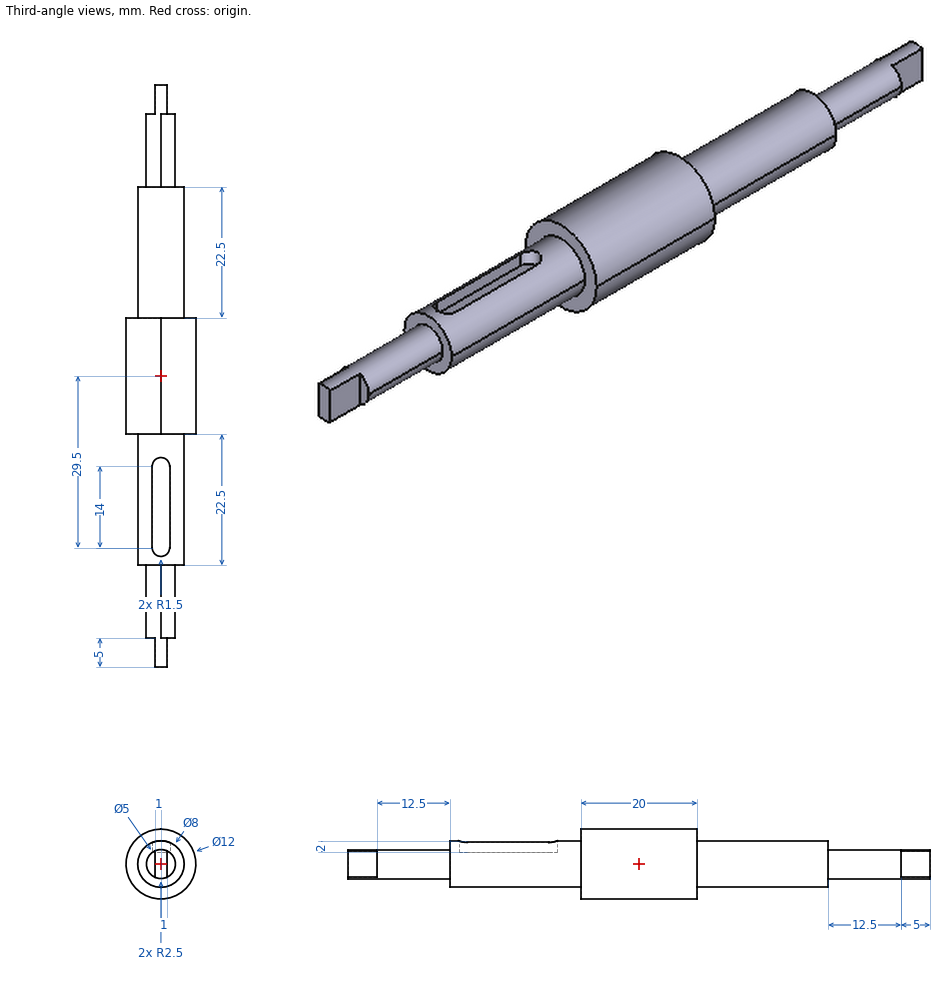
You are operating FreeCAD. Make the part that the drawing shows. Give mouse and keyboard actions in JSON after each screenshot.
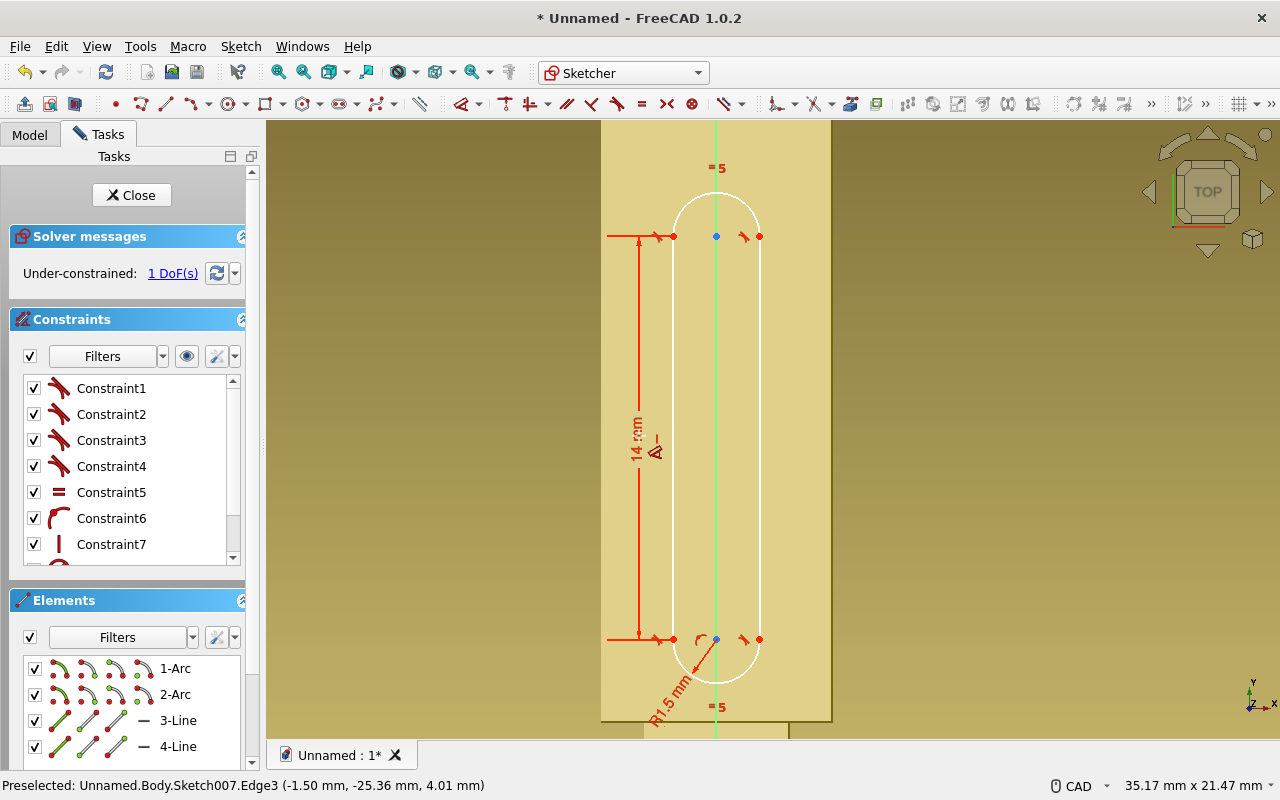
{"action": "left_click", "coordinate": [673, 640]}
{"action": "left_click", "coordinate": [639, 394]}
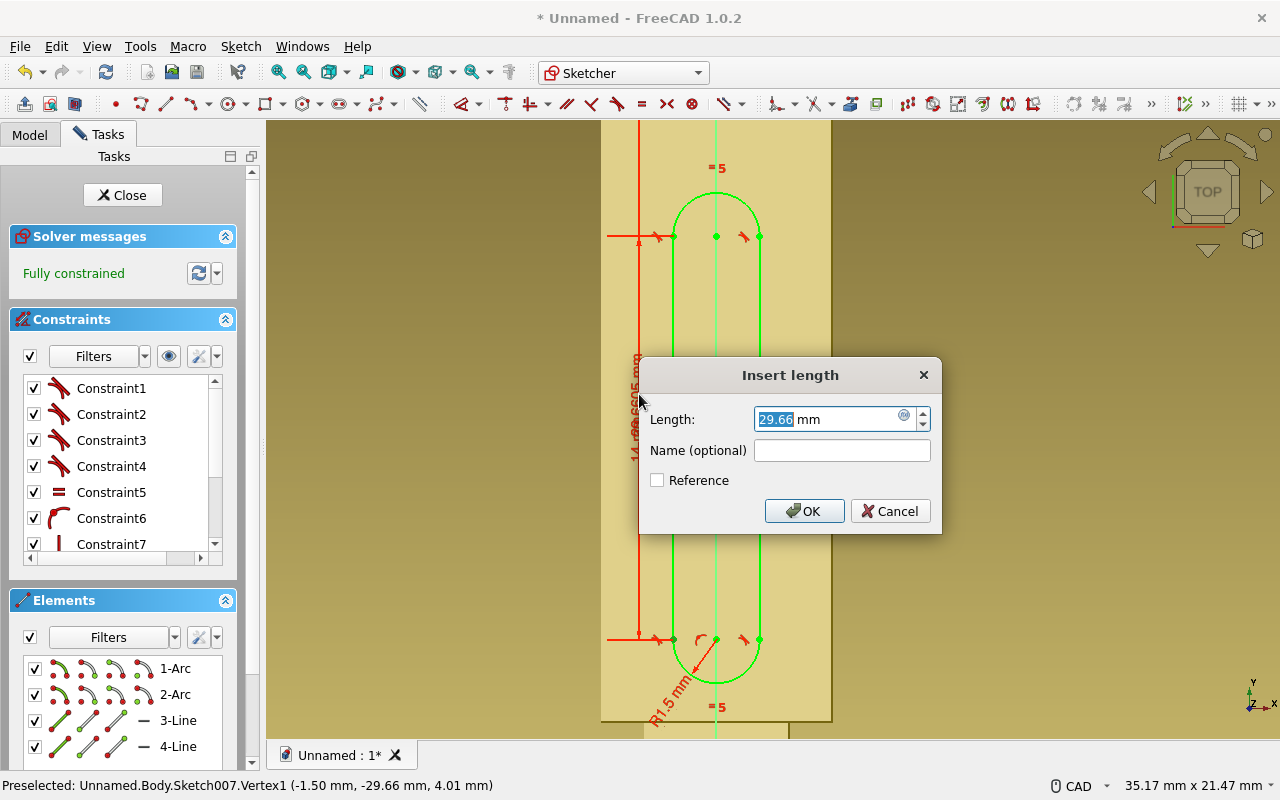
{"action": "type", "text": "29.5"}
{"action": "key", "text": "Return"}
{"action": "key", "text": "Escape"}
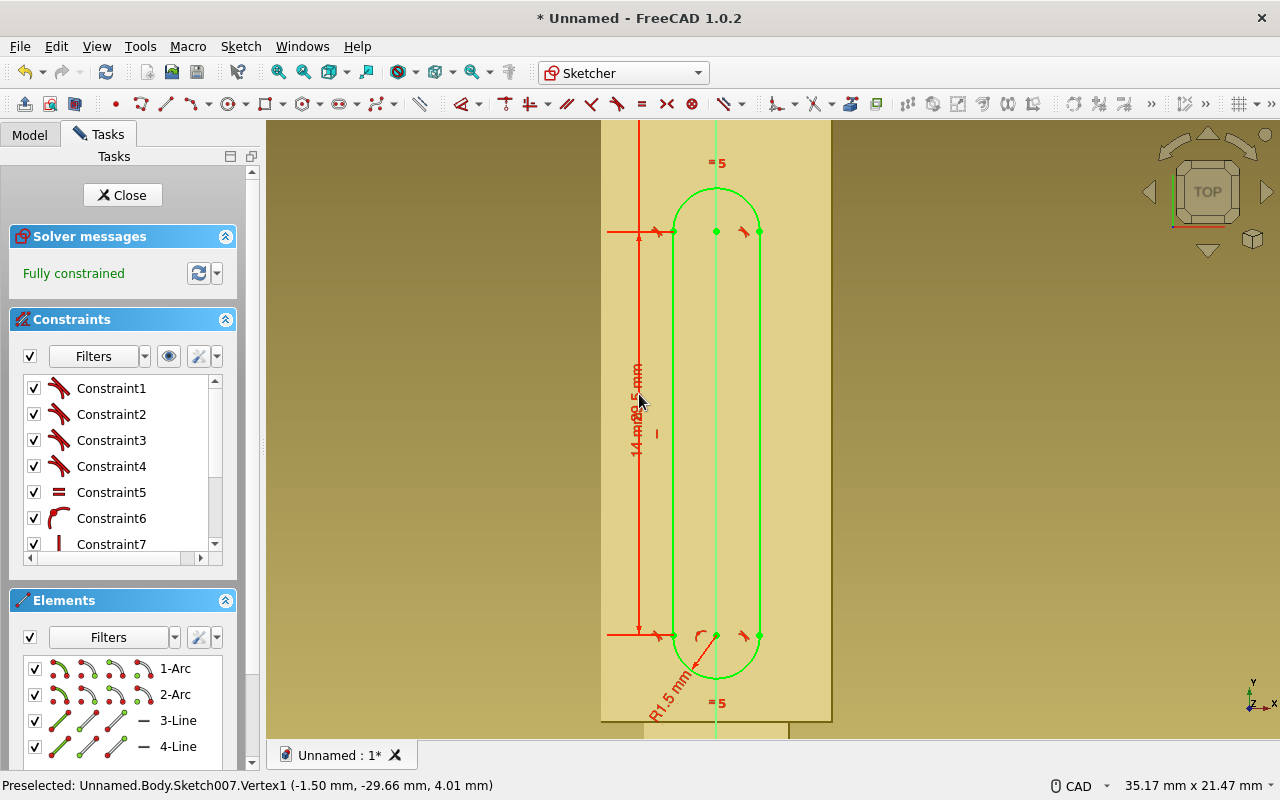
{"action": "left_click", "coordinate": [123, 195]}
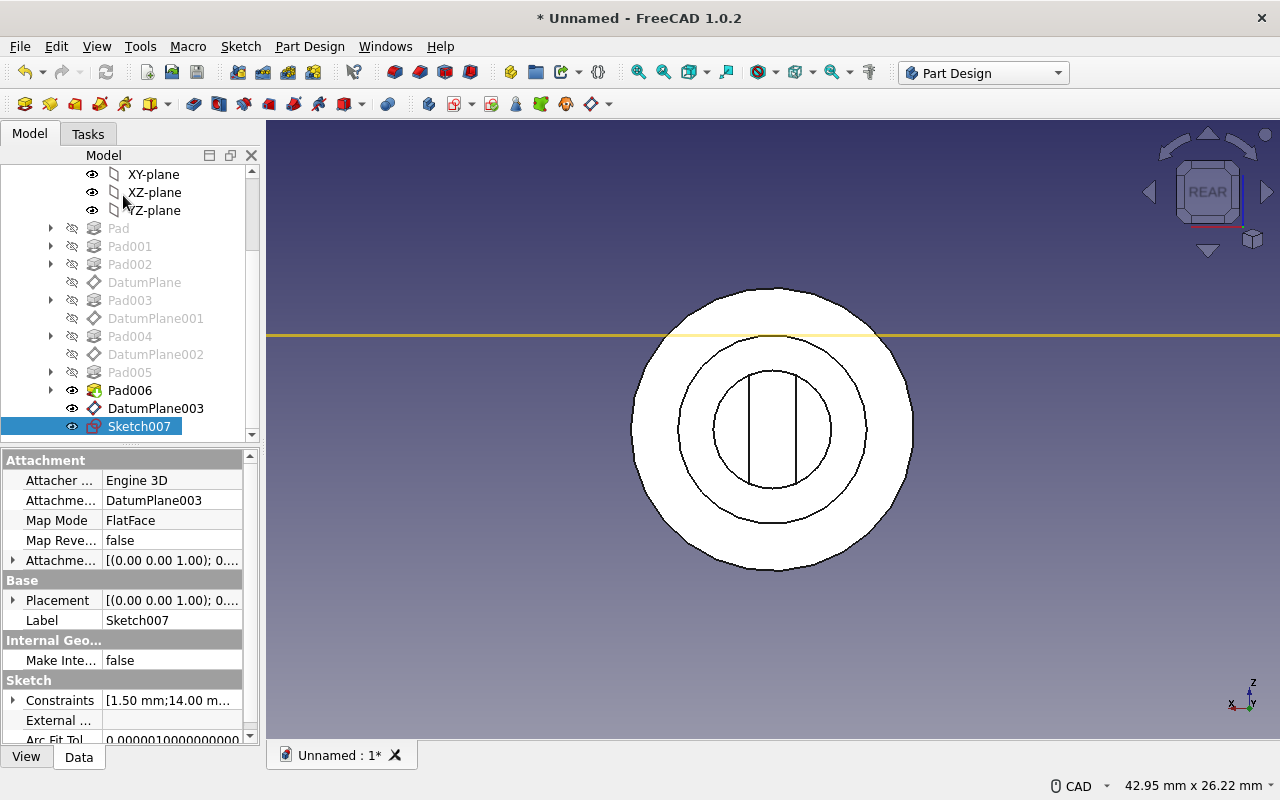
{"action": "left_click", "coordinate": [194, 104]}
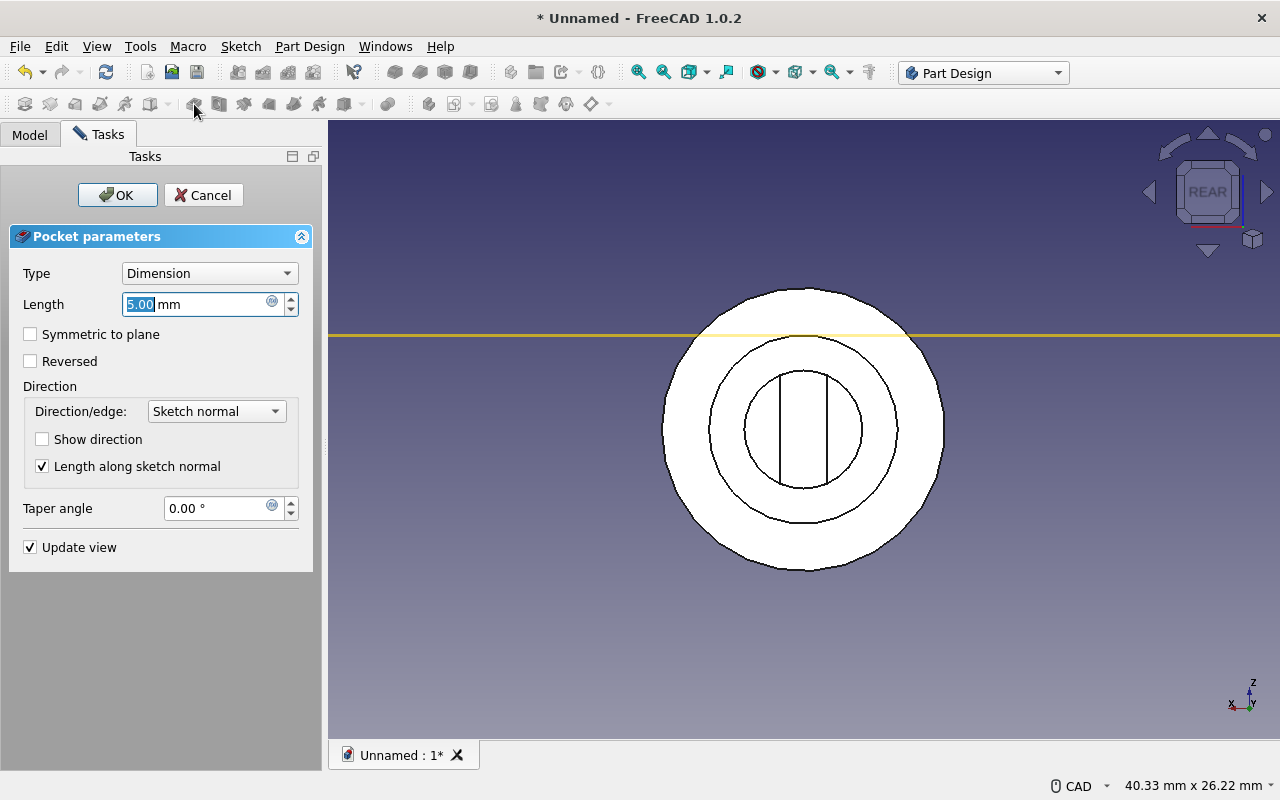
{"action": "type", "text": "2"}
{"action": "key", "text": "Tab"}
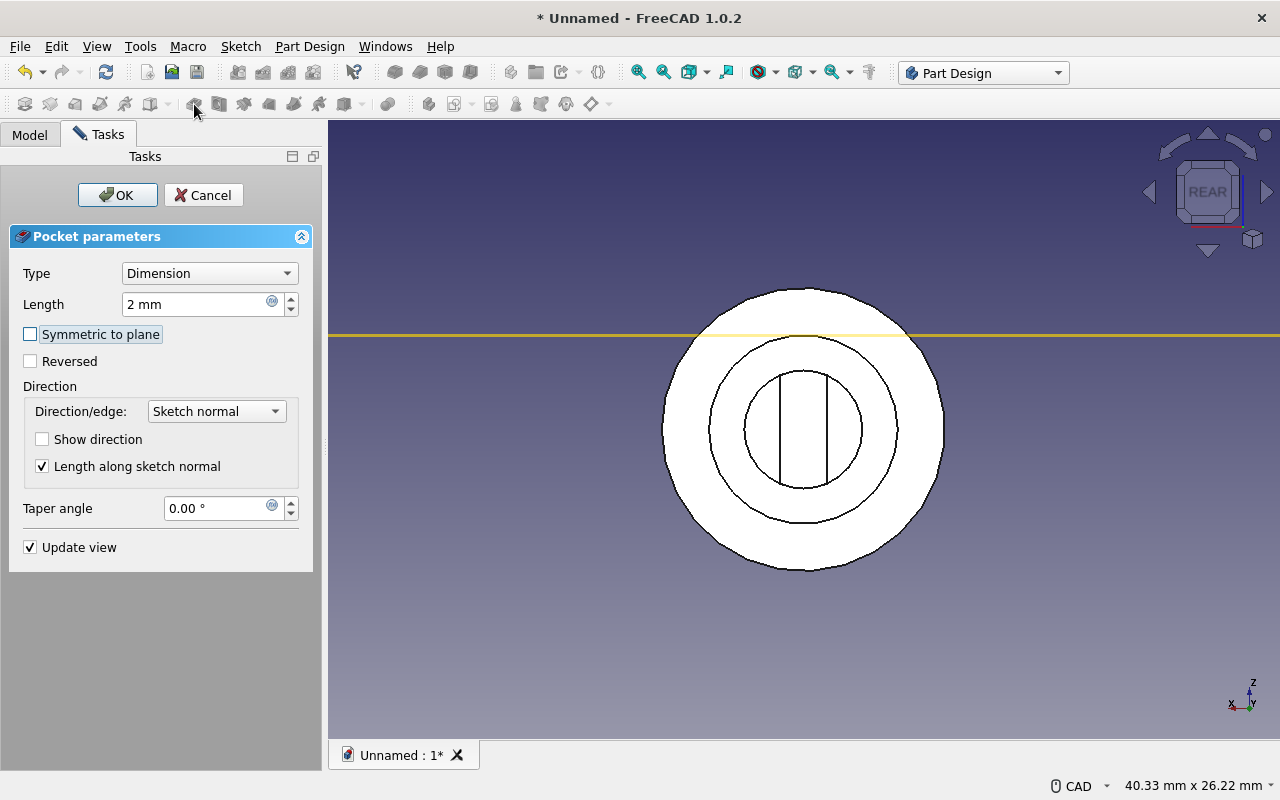
{"action": "left_click", "coordinate": [118, 195]}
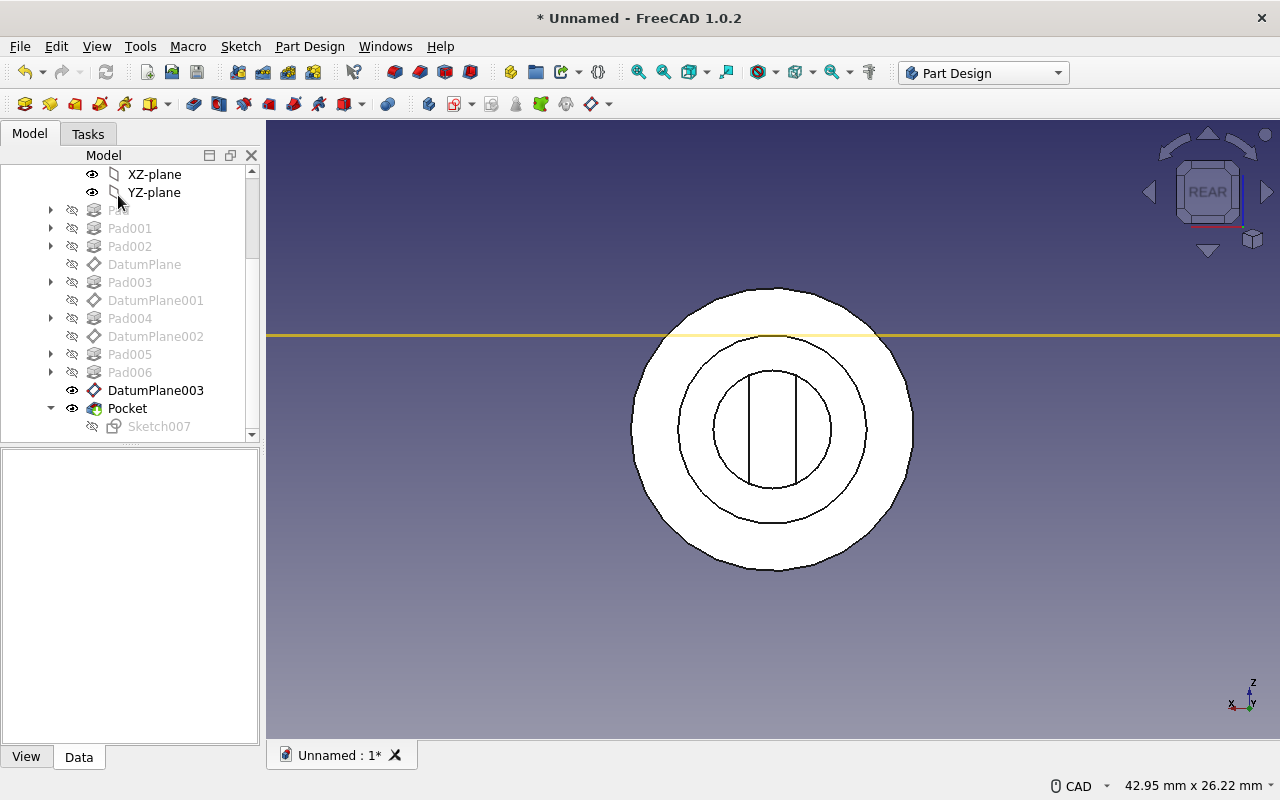
{"action": "left_click", "coordinate": [117, 390]}
{"action": "key", "text": "space"}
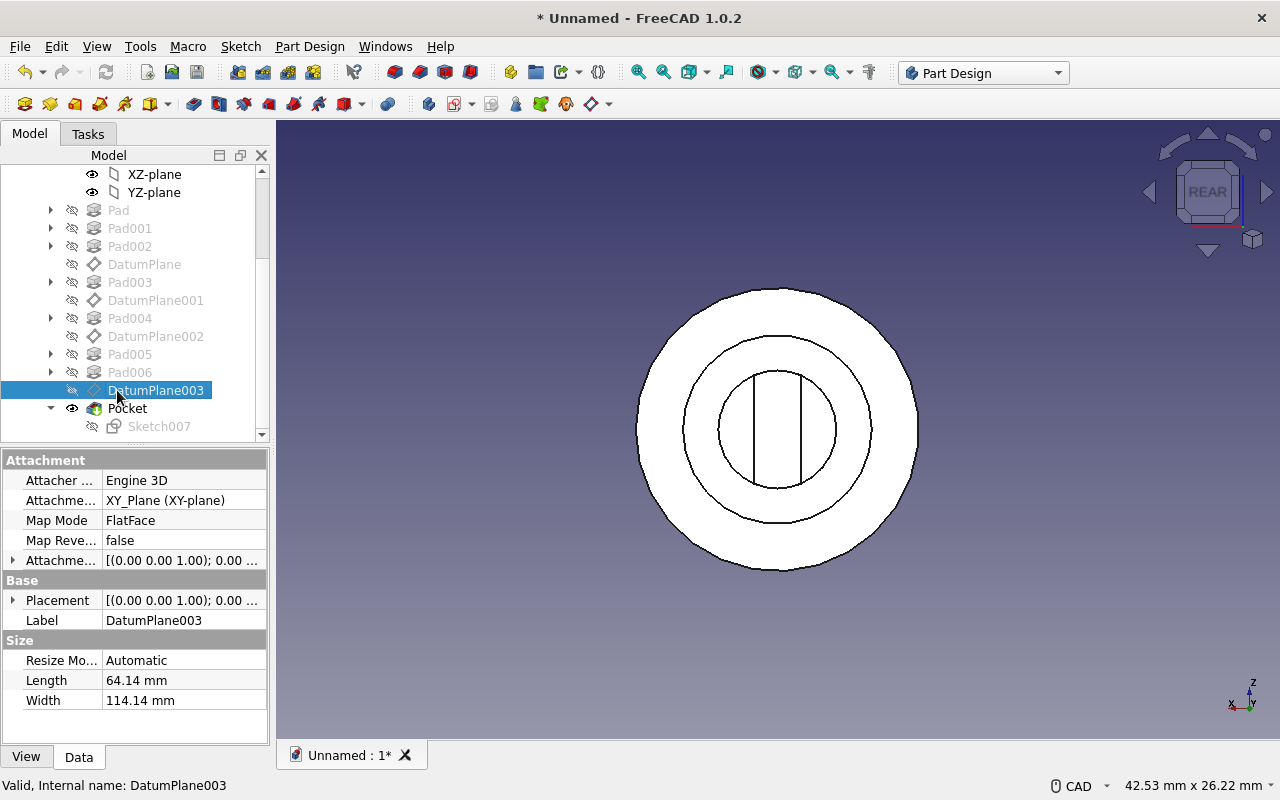
{"action": "key", "text": "0"}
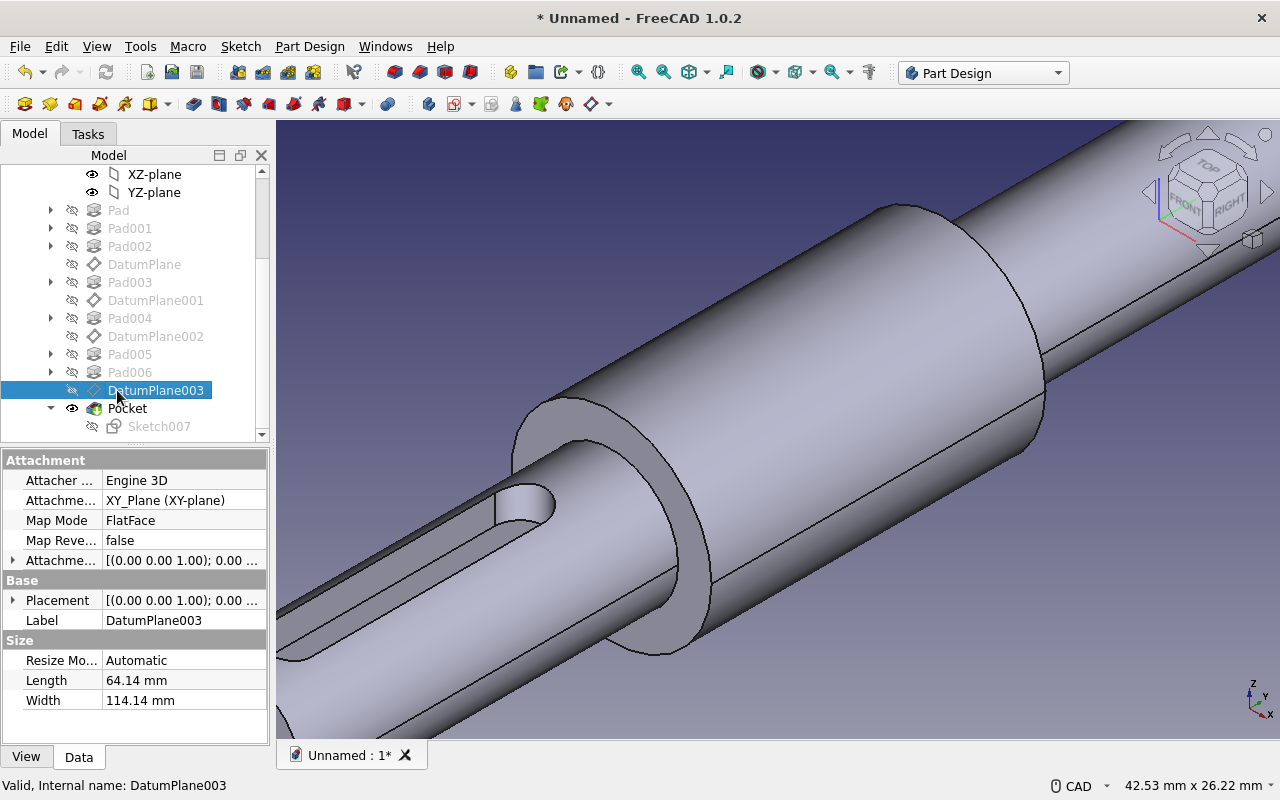
{"action": "key", "text": "v f"}